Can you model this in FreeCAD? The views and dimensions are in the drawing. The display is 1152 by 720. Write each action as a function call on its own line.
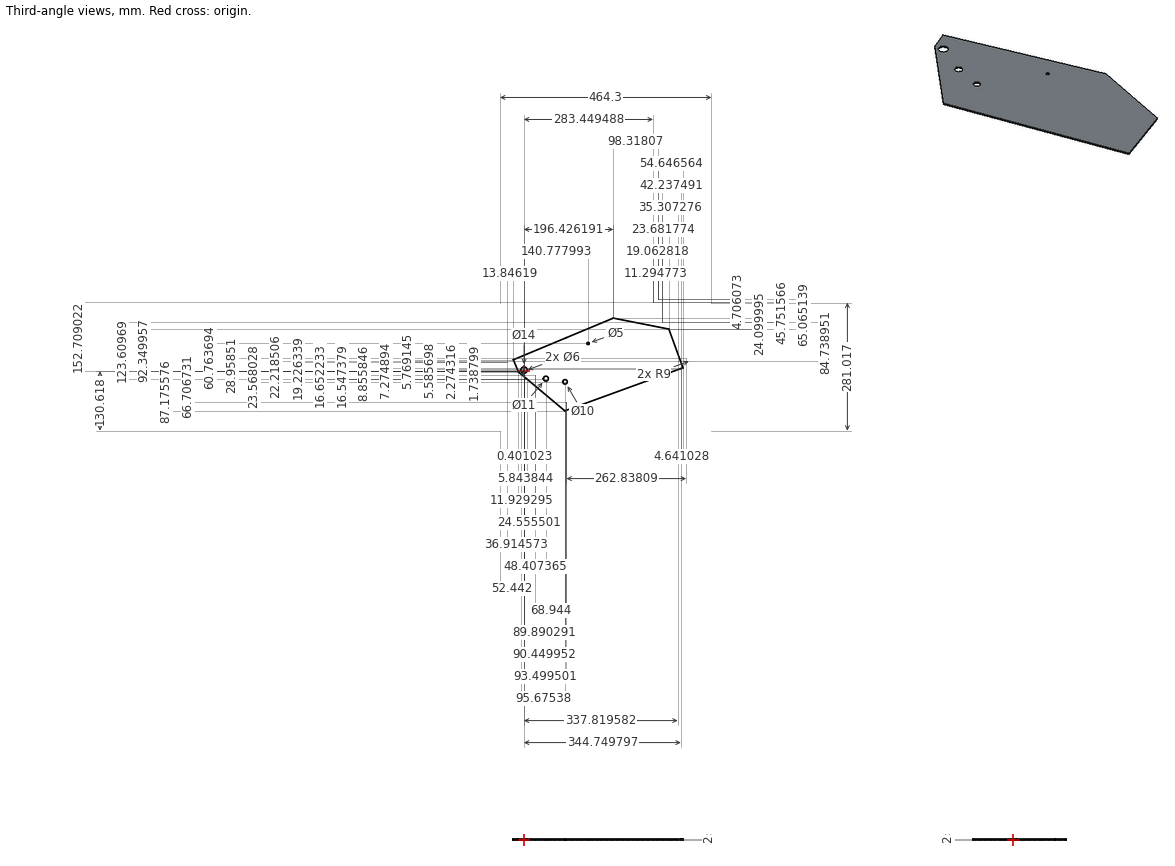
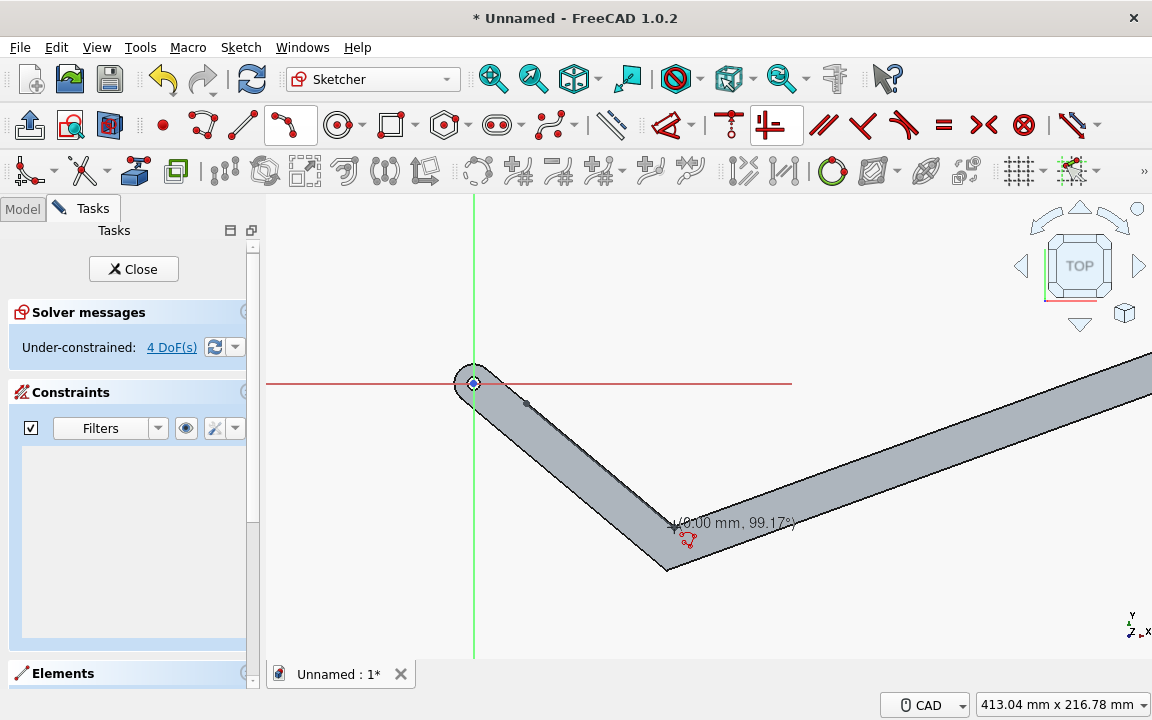
scroll(294, 602, down, 2)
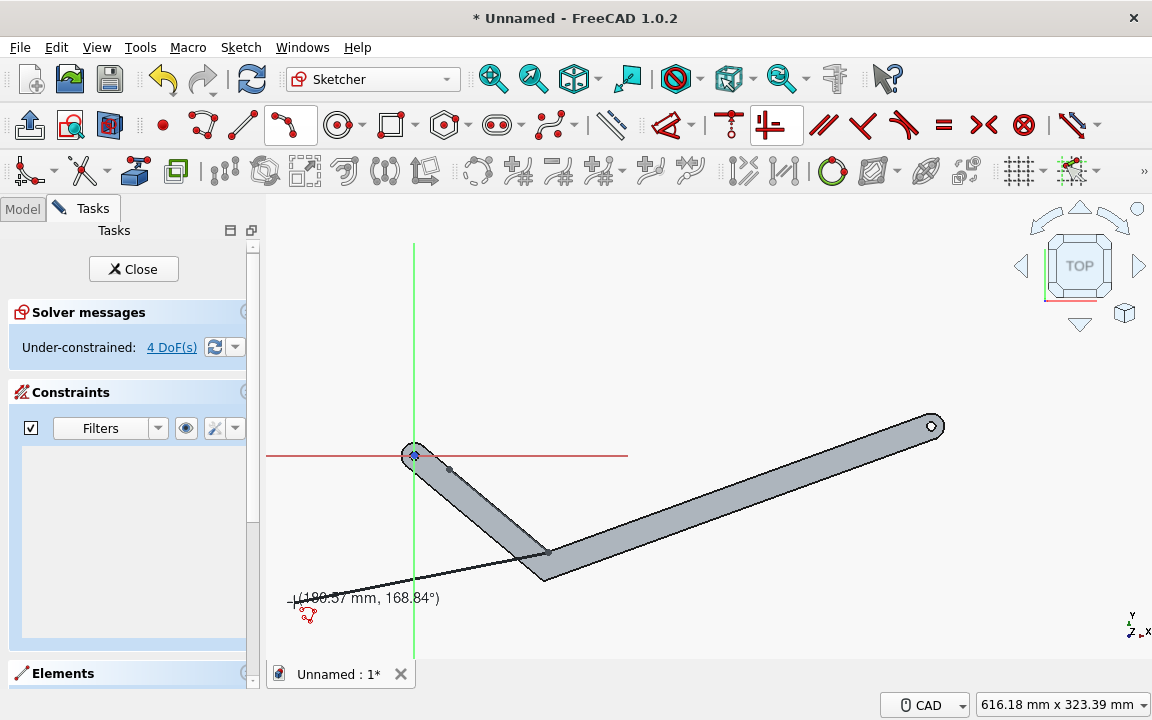
click(900, 424)
click(849, 302)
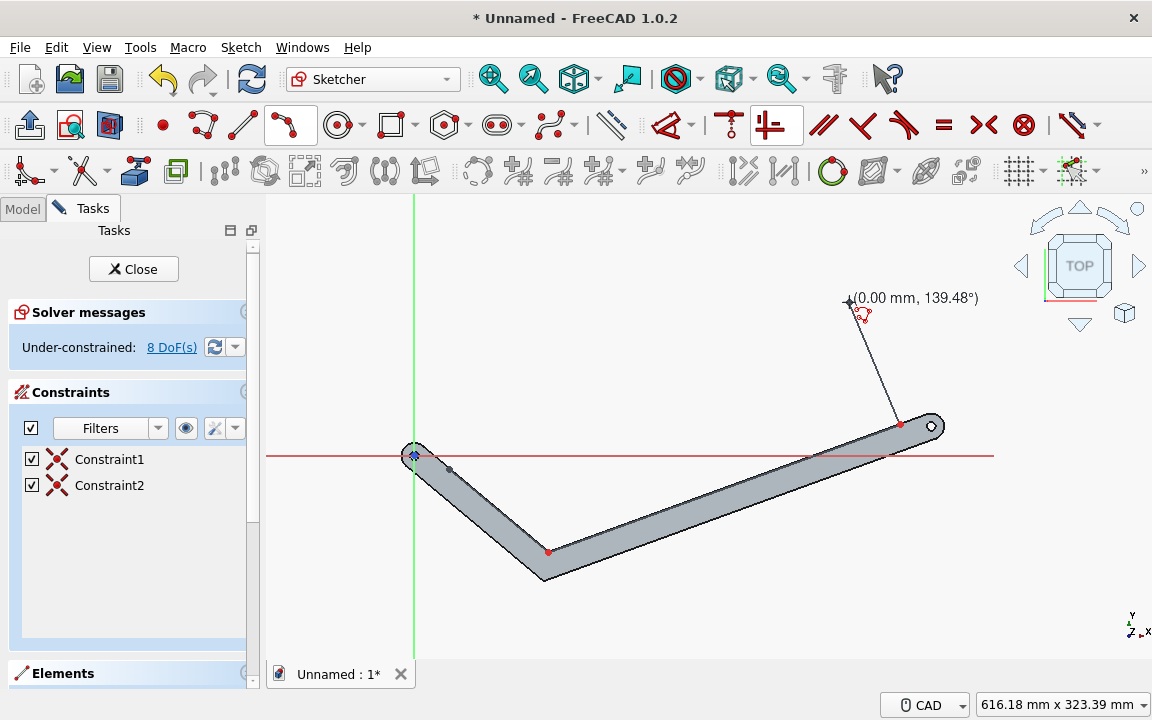
scroll(450, 469, up, 2)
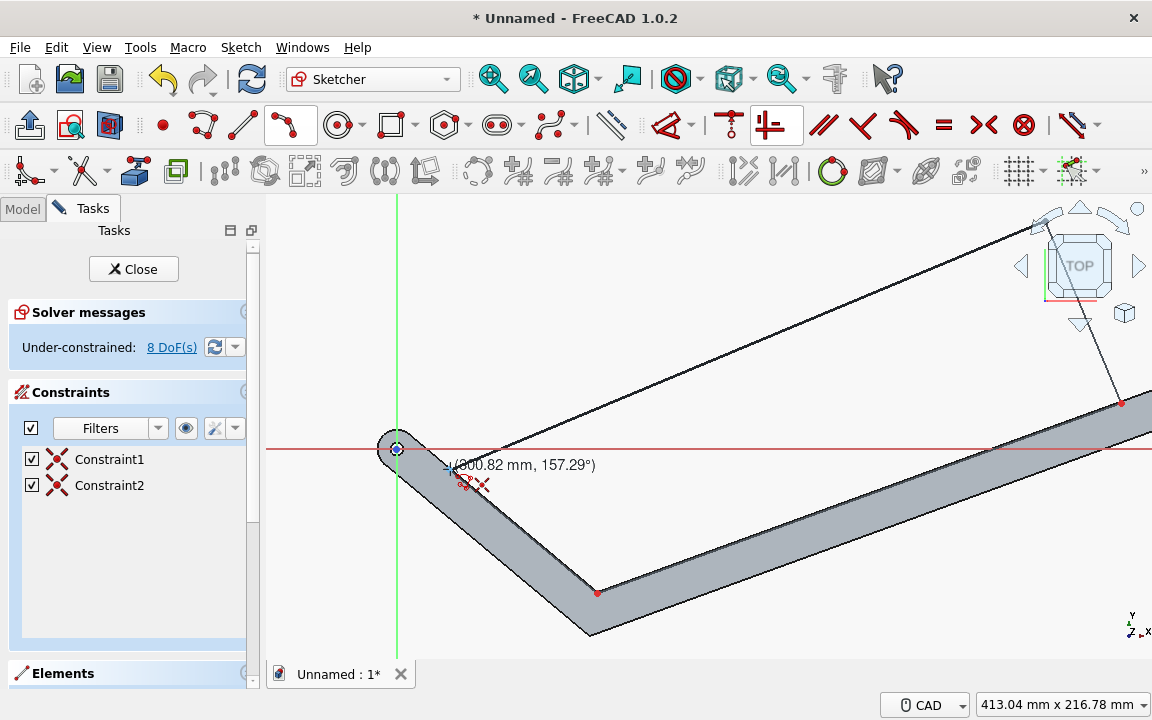
click(449, 470)
key(Escape)
key(Escape)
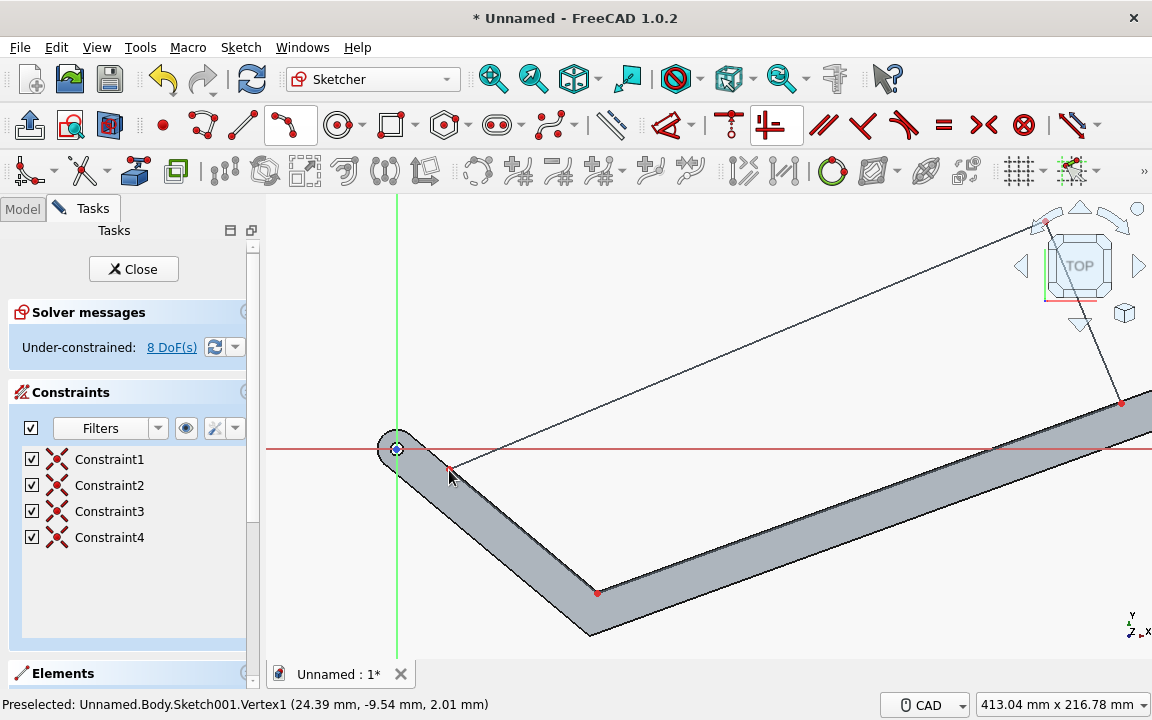
click(494, 507)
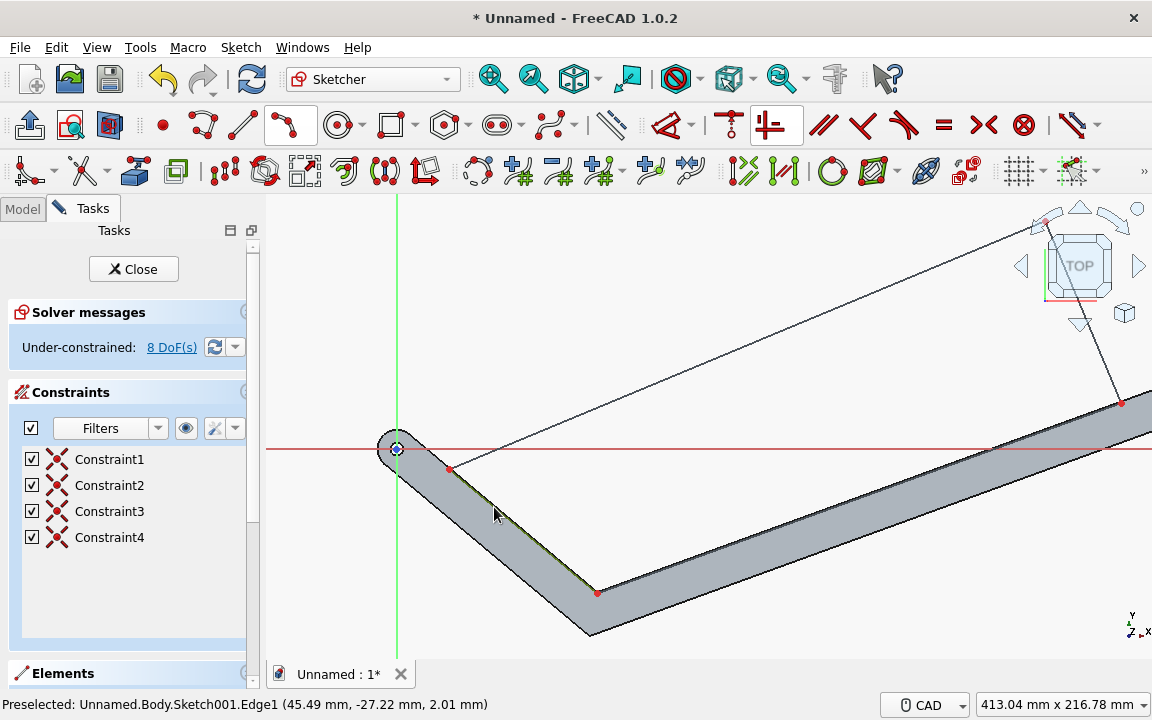
key(l)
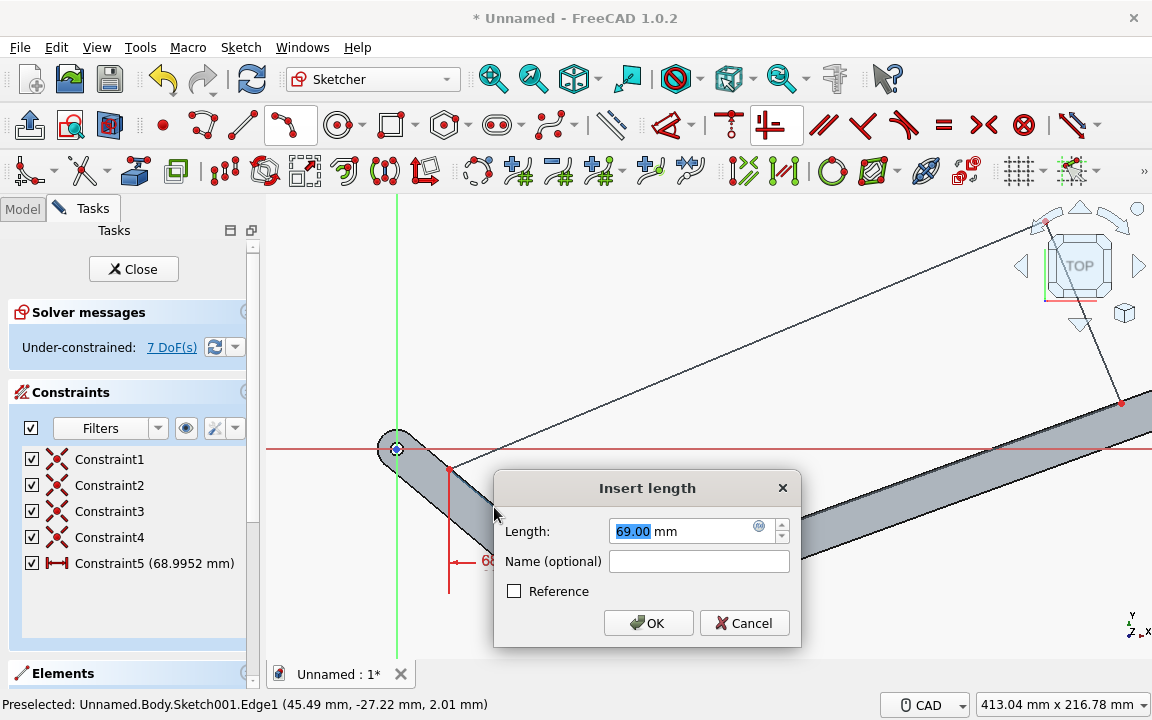
text(68.944)
key(Return)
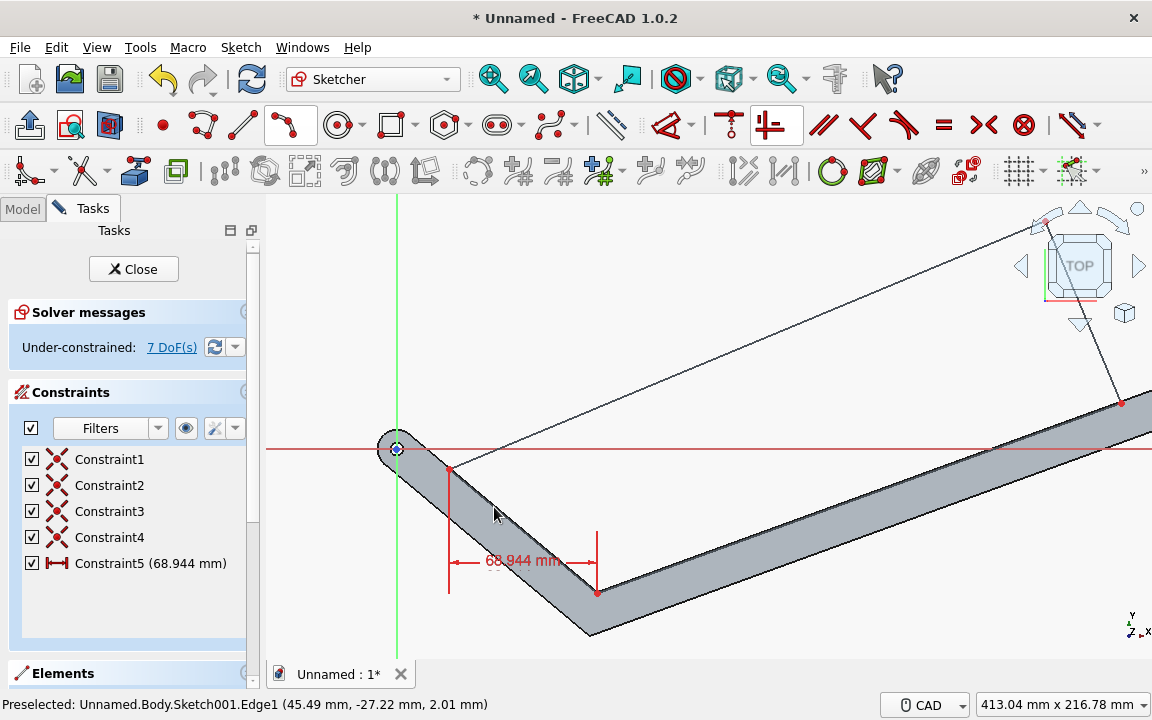
scroll(449, 470, up, 4)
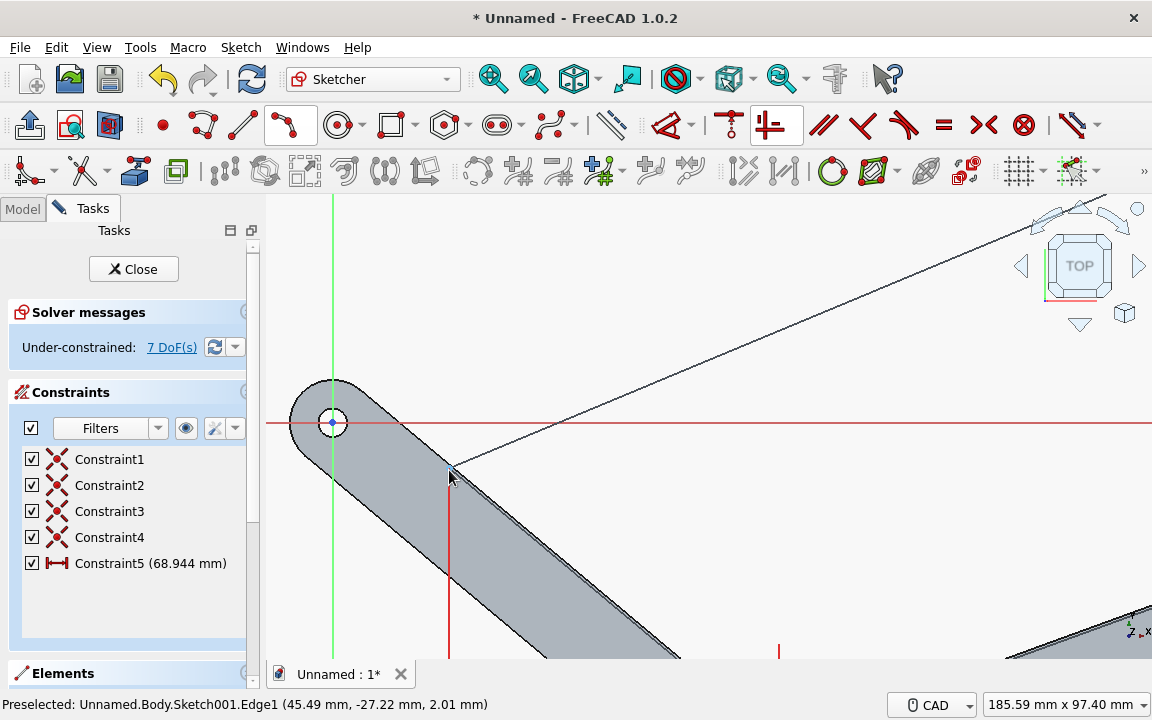
click(449, 468)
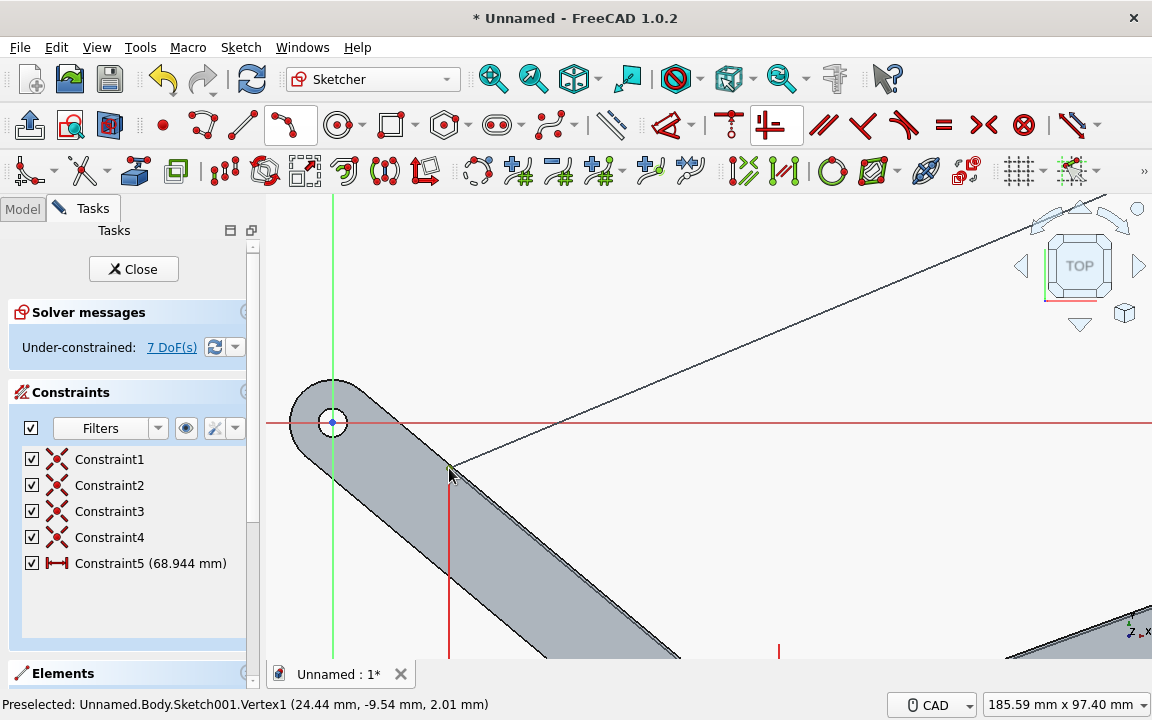
key(i)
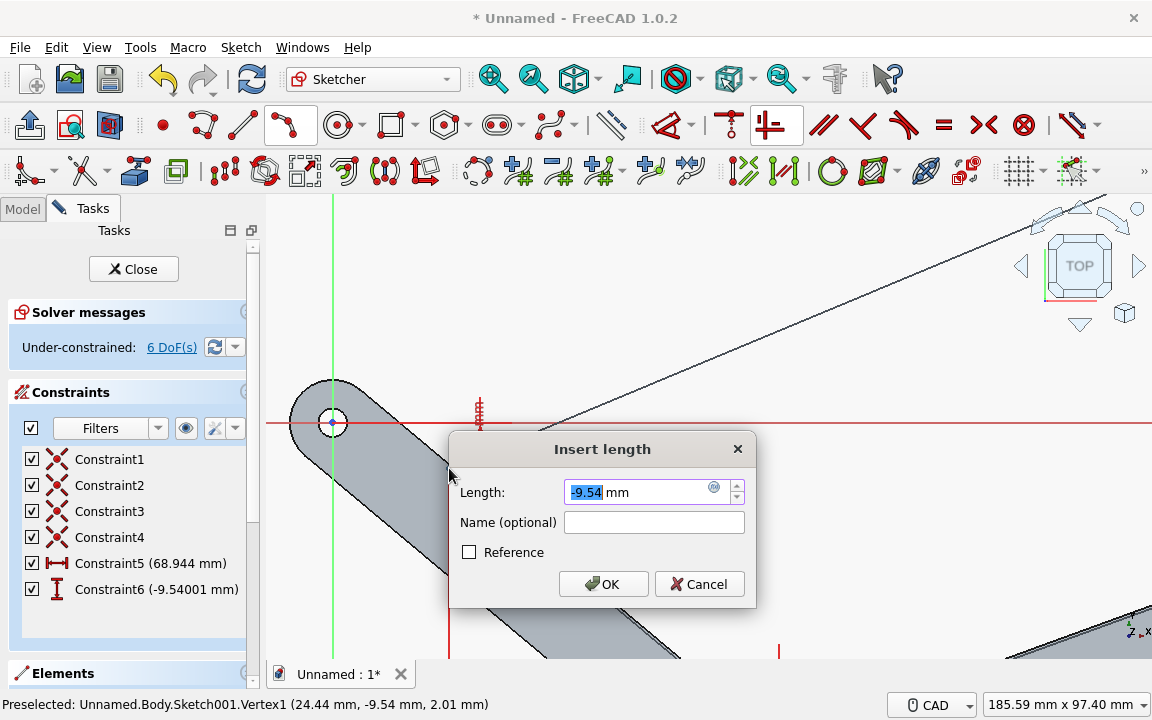
text(-8.855846)
key(Return)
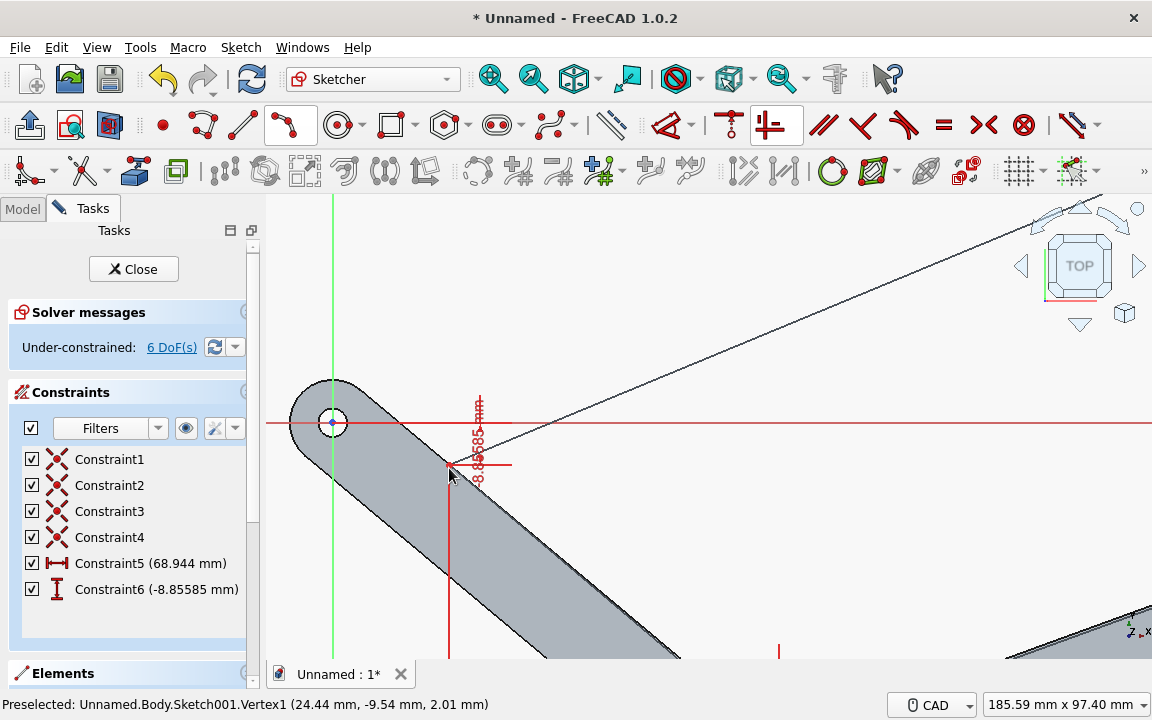
scroll(426, 470, down, 6)